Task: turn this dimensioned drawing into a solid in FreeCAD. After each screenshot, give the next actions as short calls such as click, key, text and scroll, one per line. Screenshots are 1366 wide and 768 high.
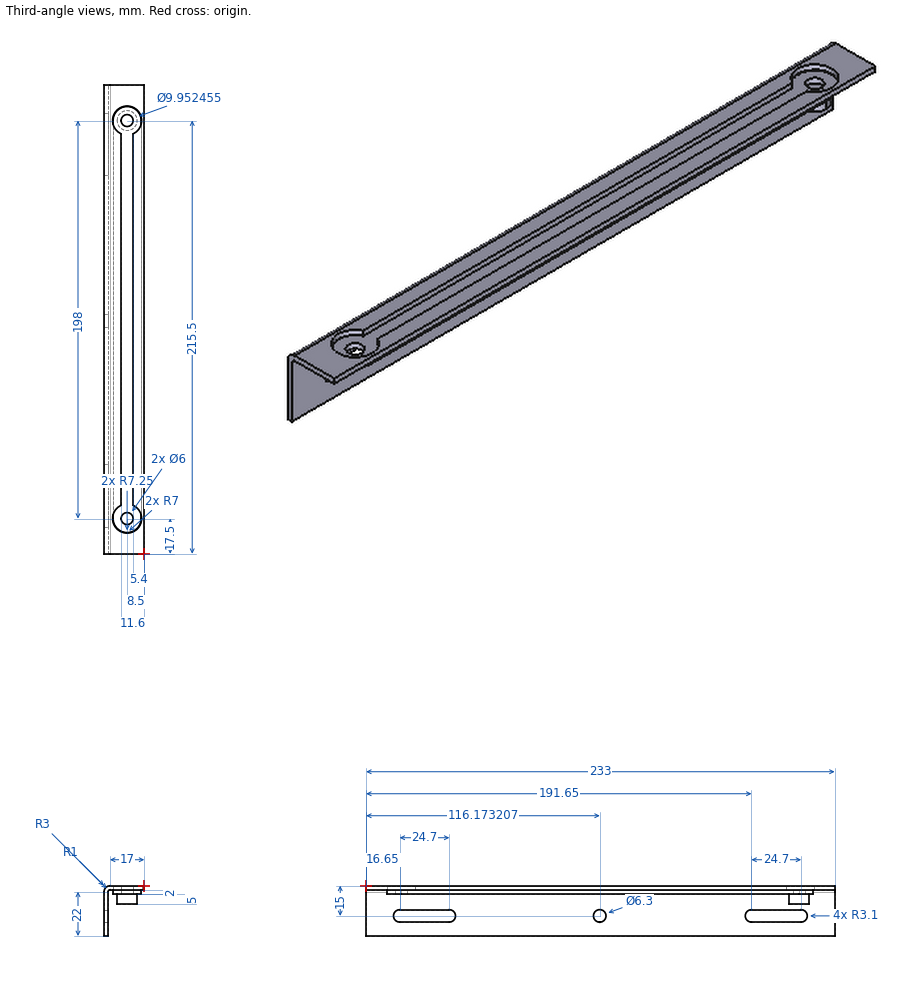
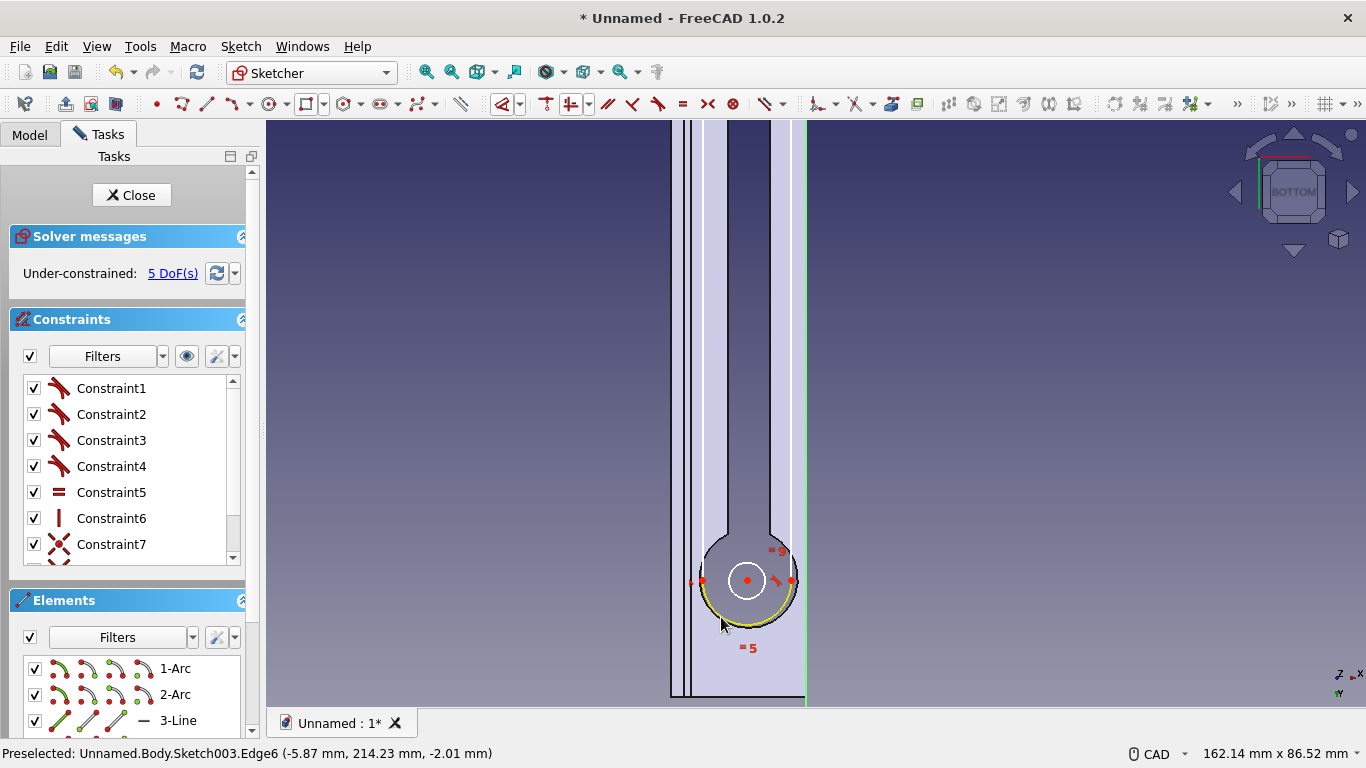
click(721, 617)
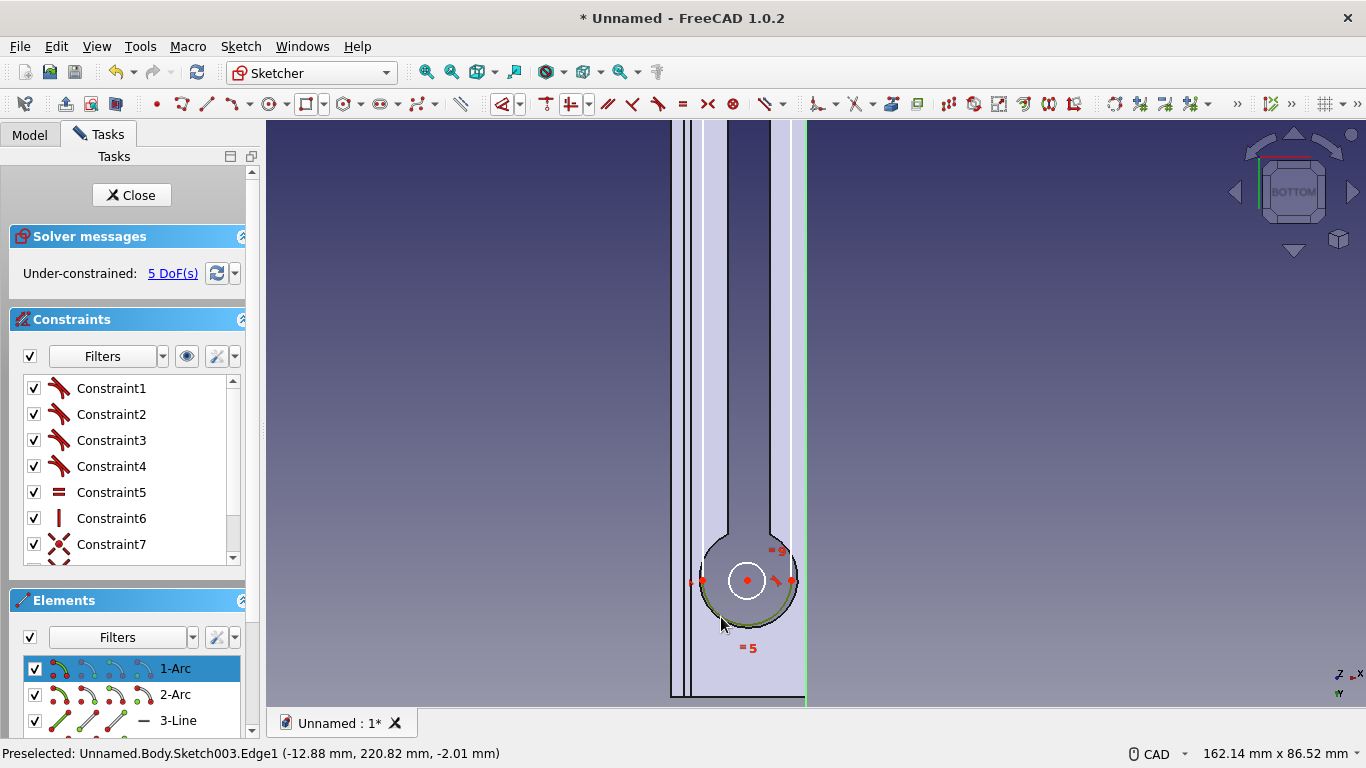
key(k)
key(r)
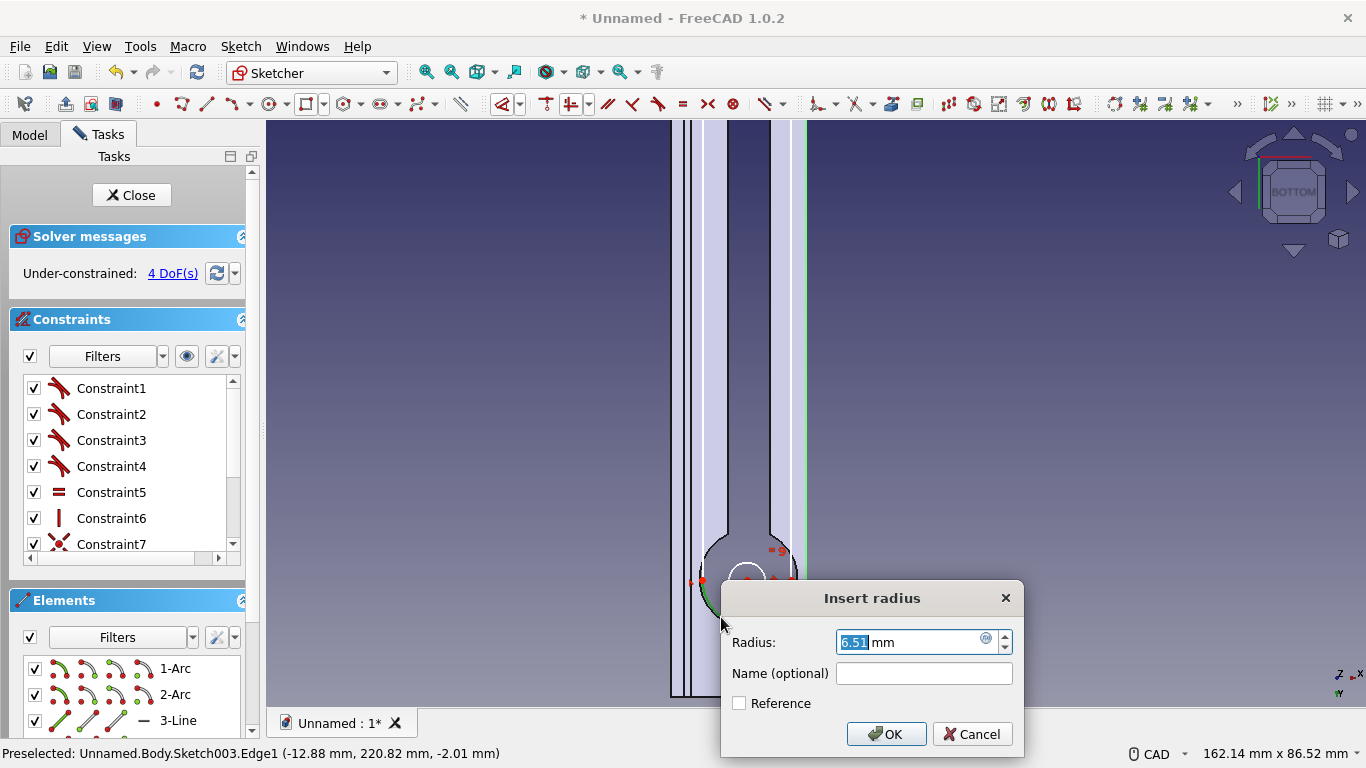
text(7)
key(Return)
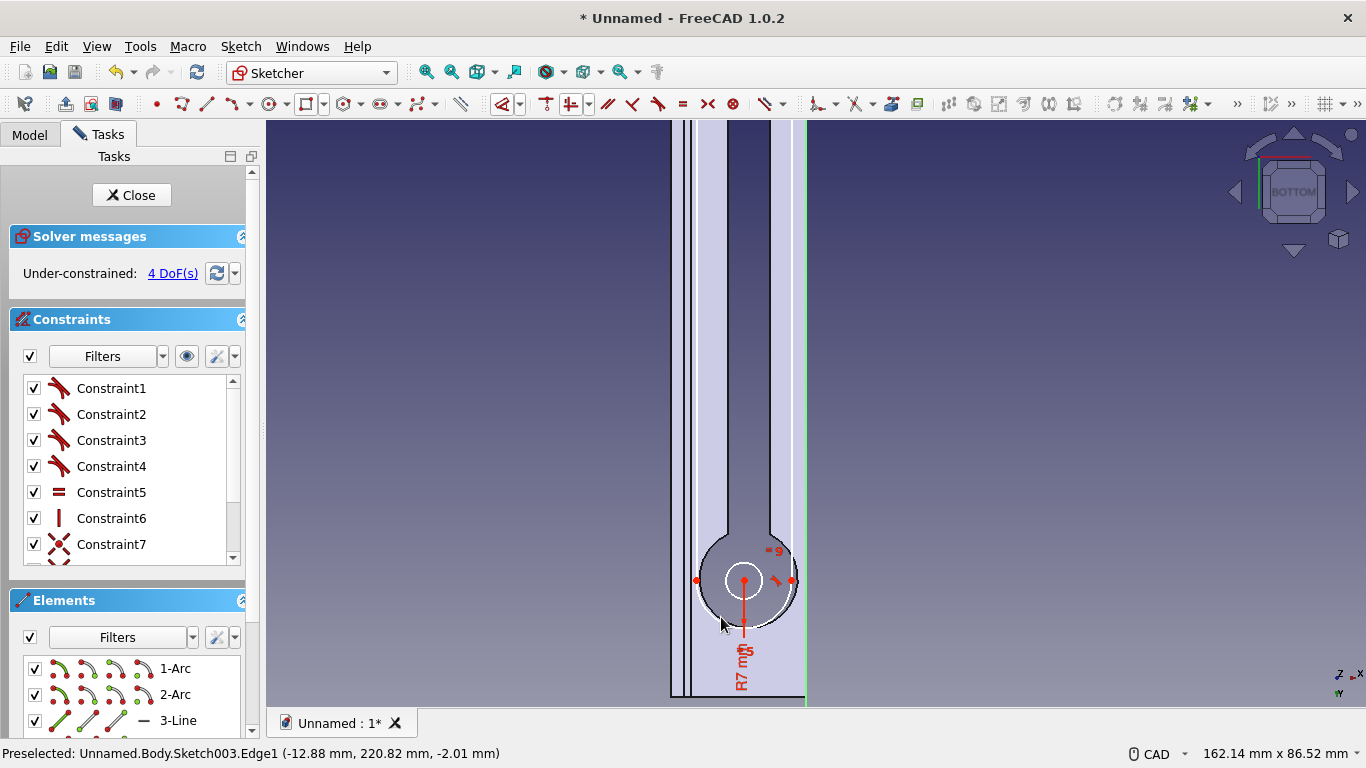
scroll(745, 591, down, 7)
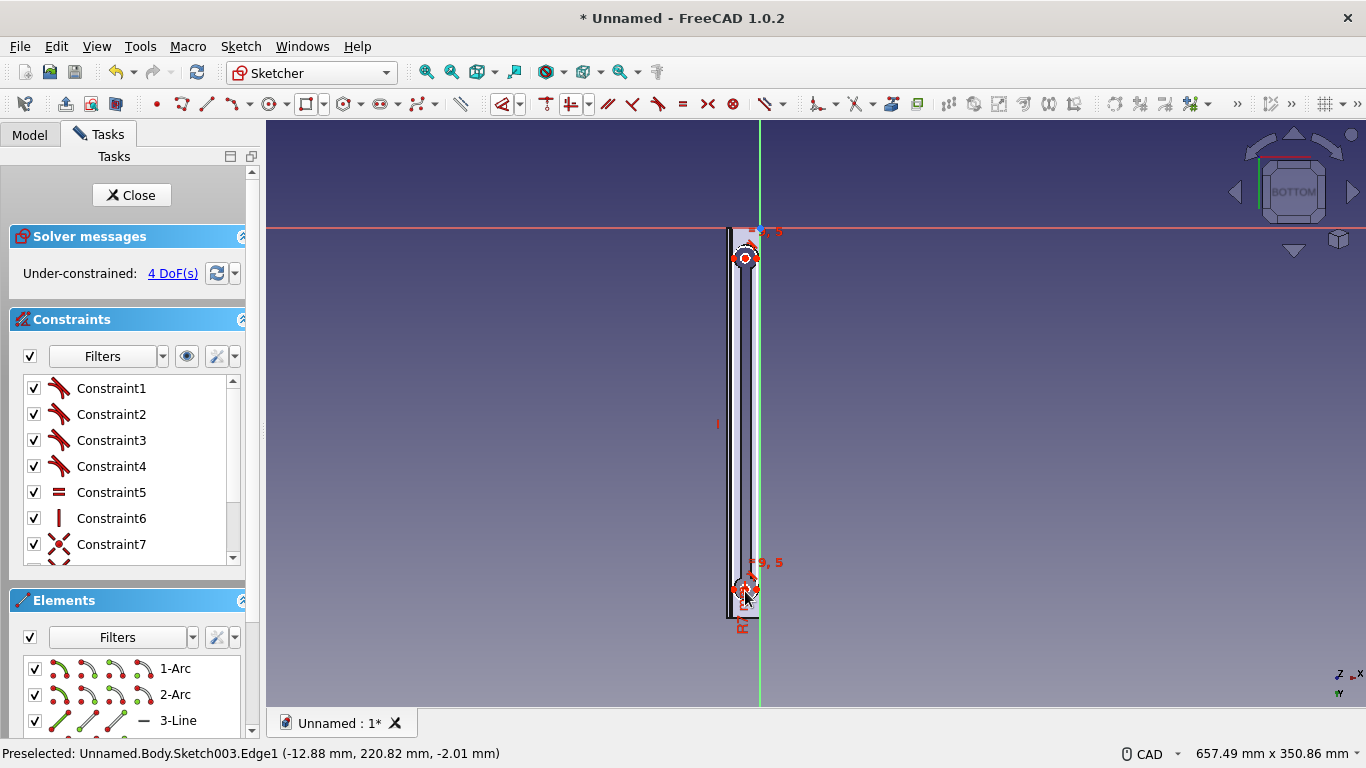
scroll(748, 255, up, 7)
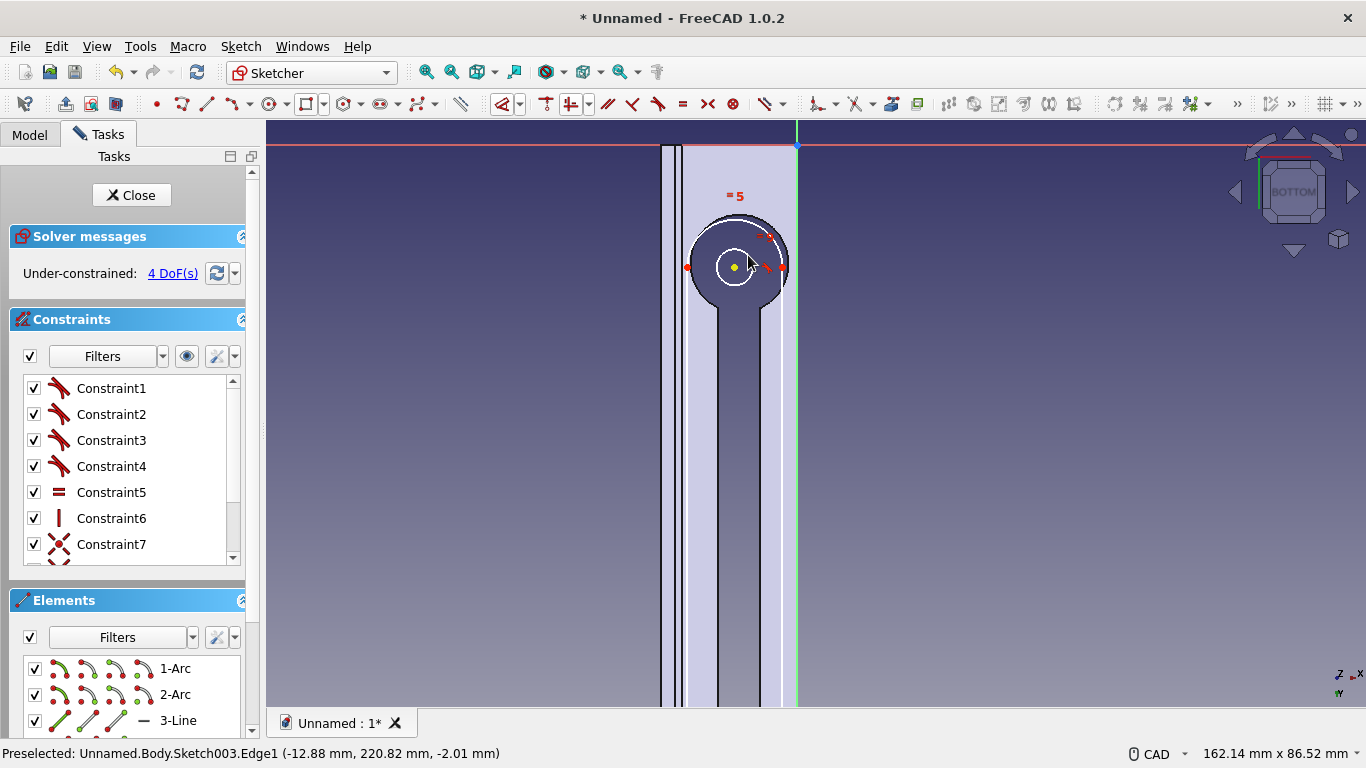
click(748, 255)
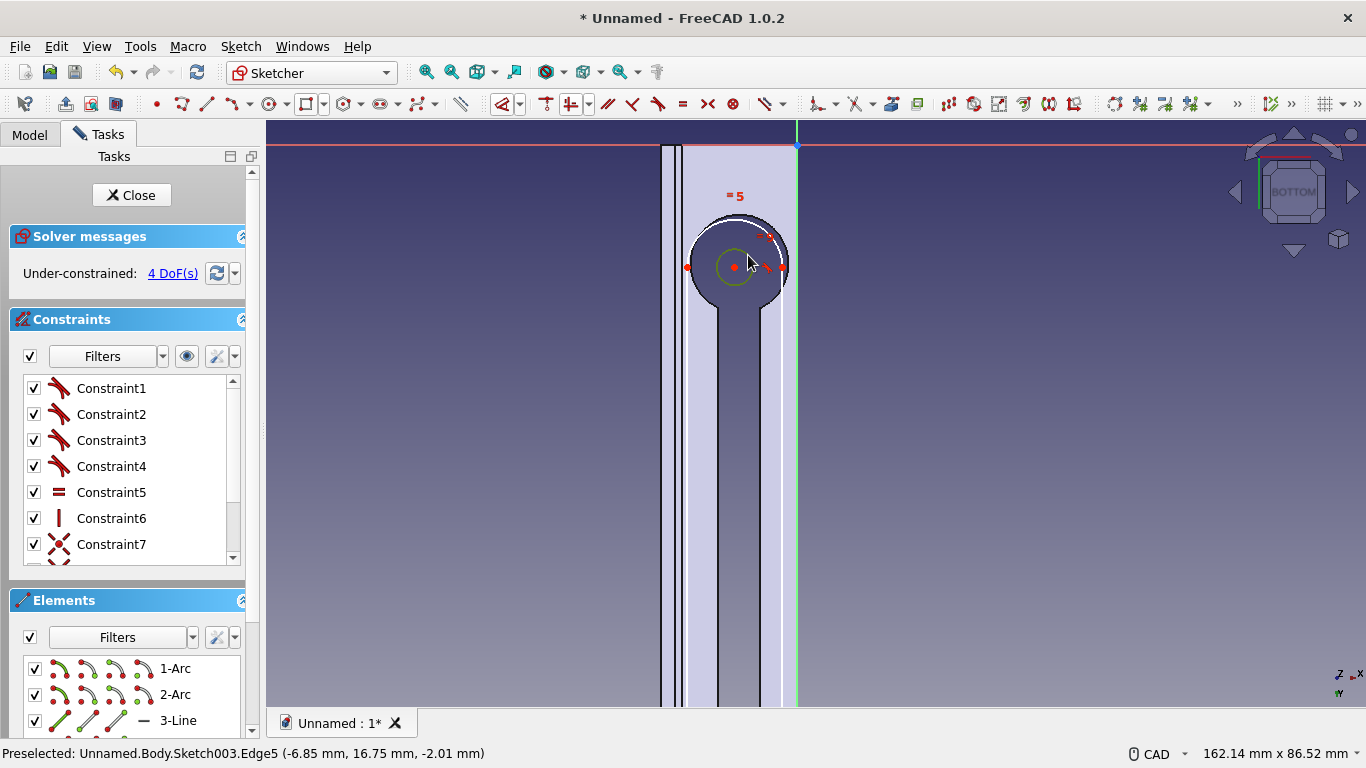
click(520, 104)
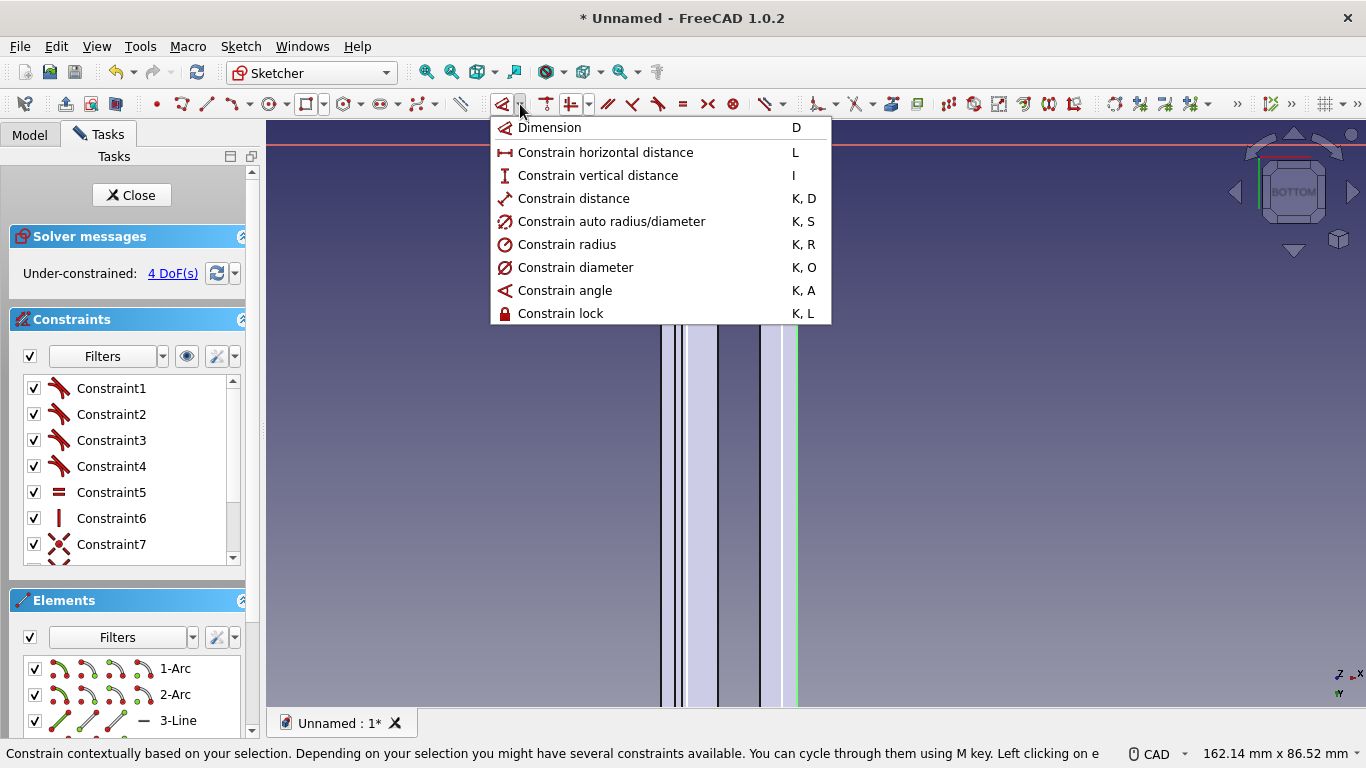
click(661, 268)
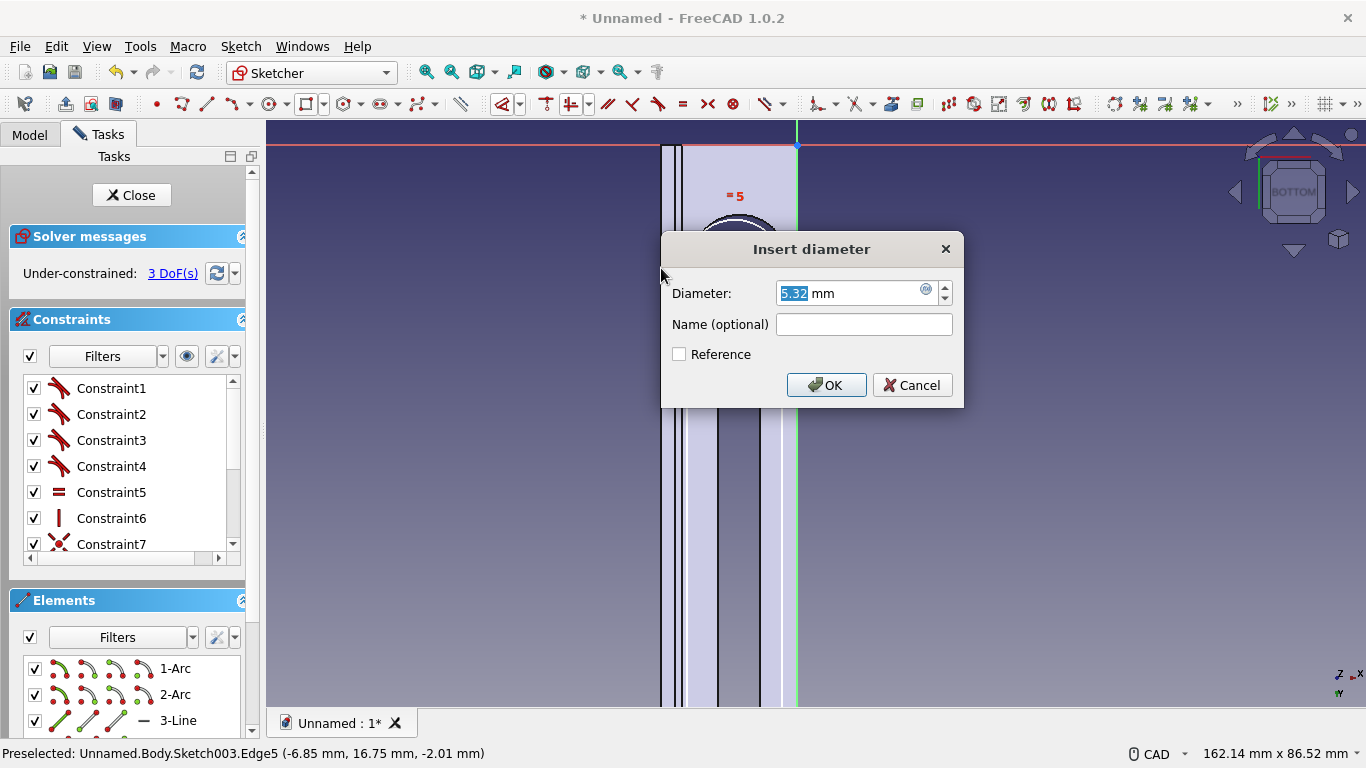
text(6)
key(Return)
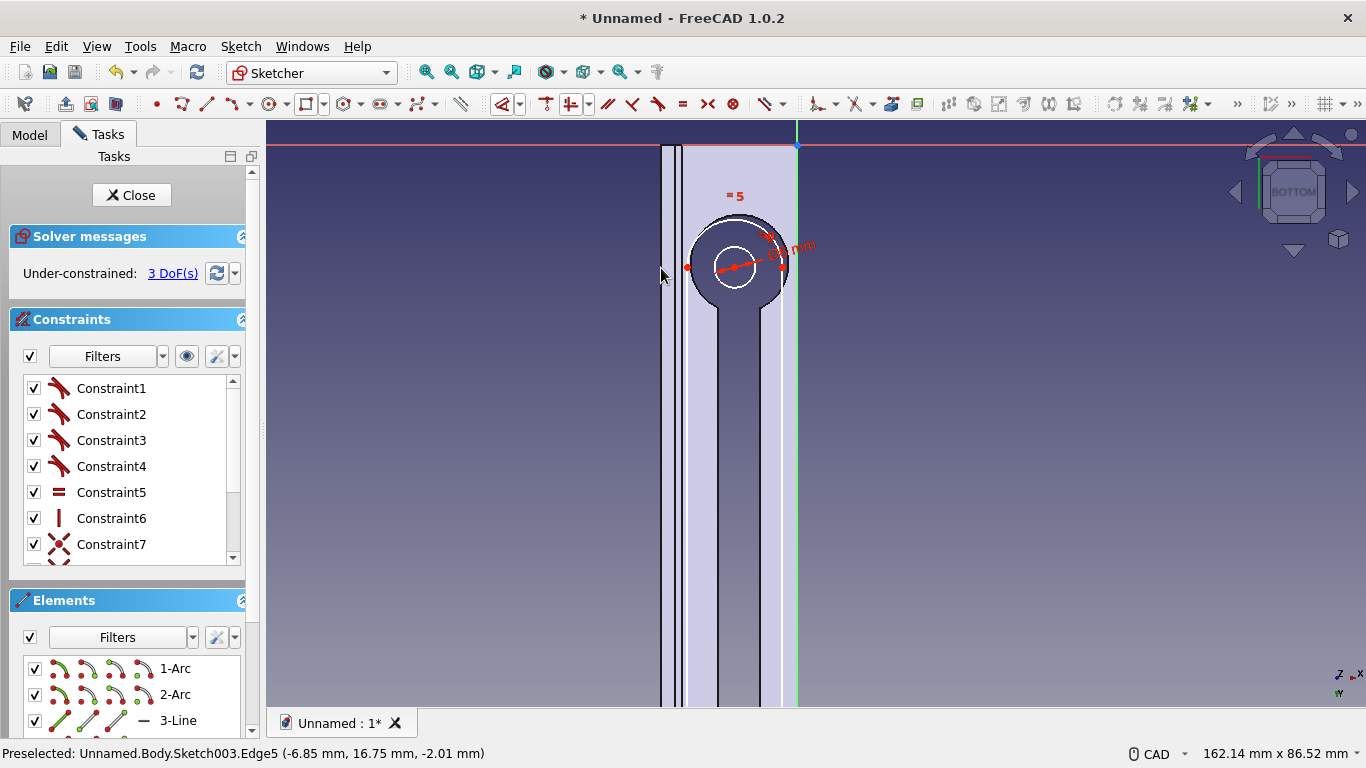
scroll(748, 254, down, 7)